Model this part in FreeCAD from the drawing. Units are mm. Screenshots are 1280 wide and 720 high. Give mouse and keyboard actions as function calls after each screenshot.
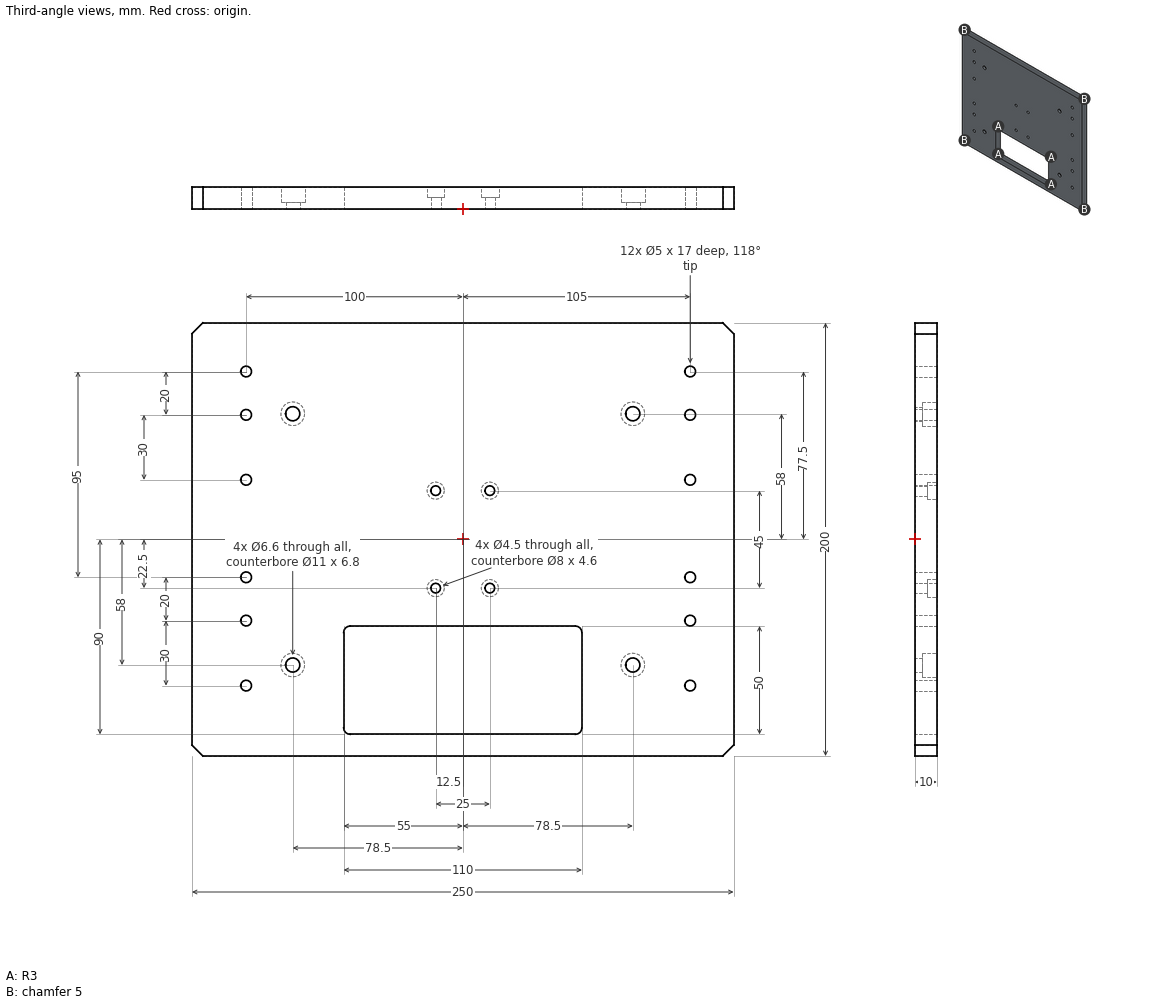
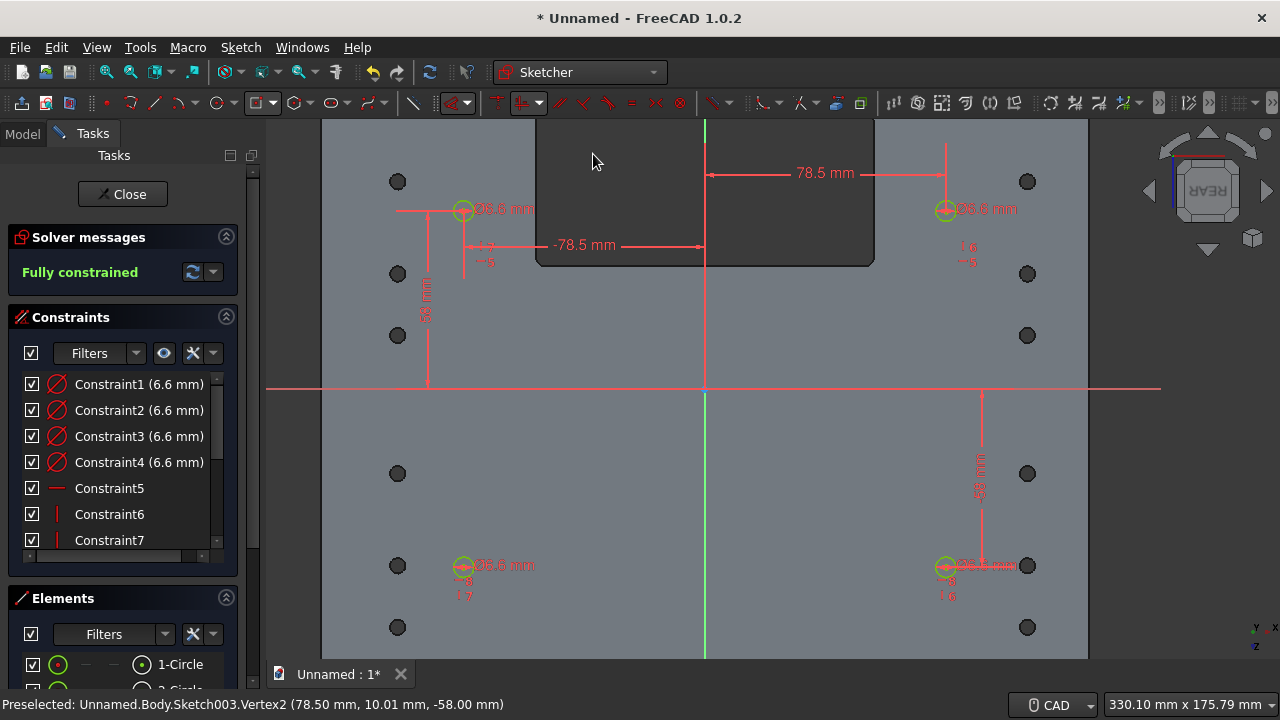
click(123, 194)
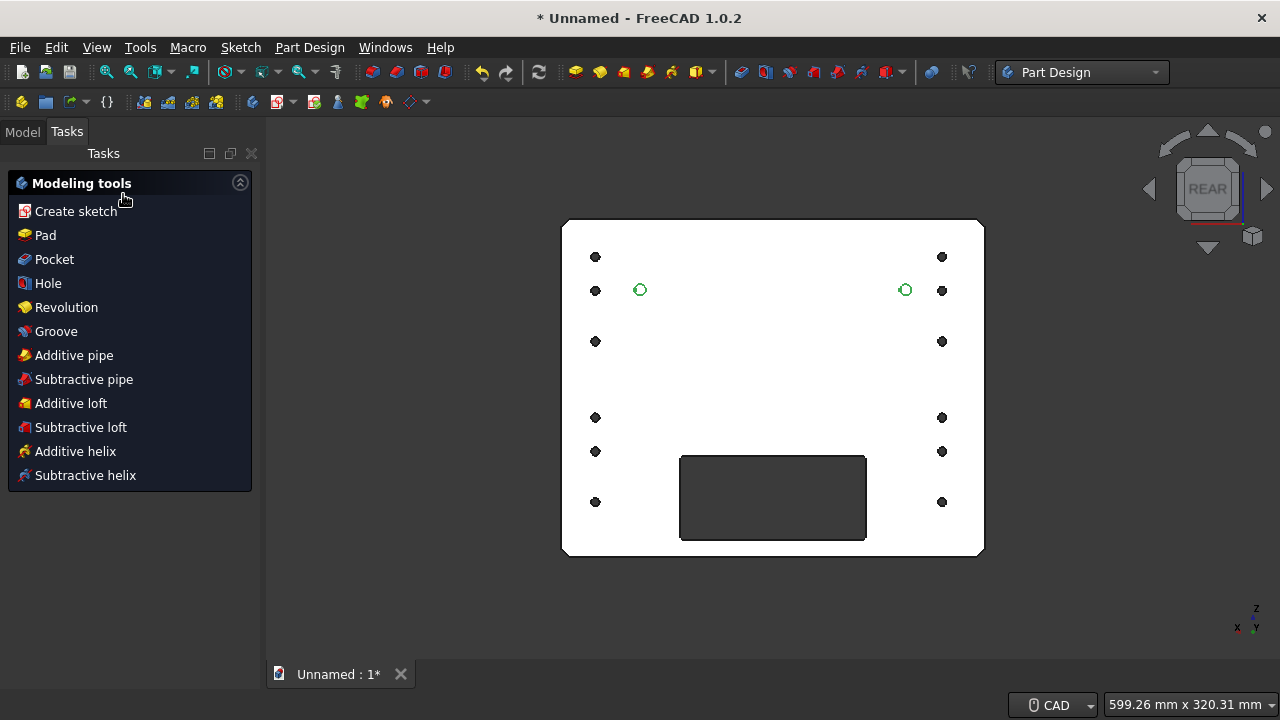
click(766, 72)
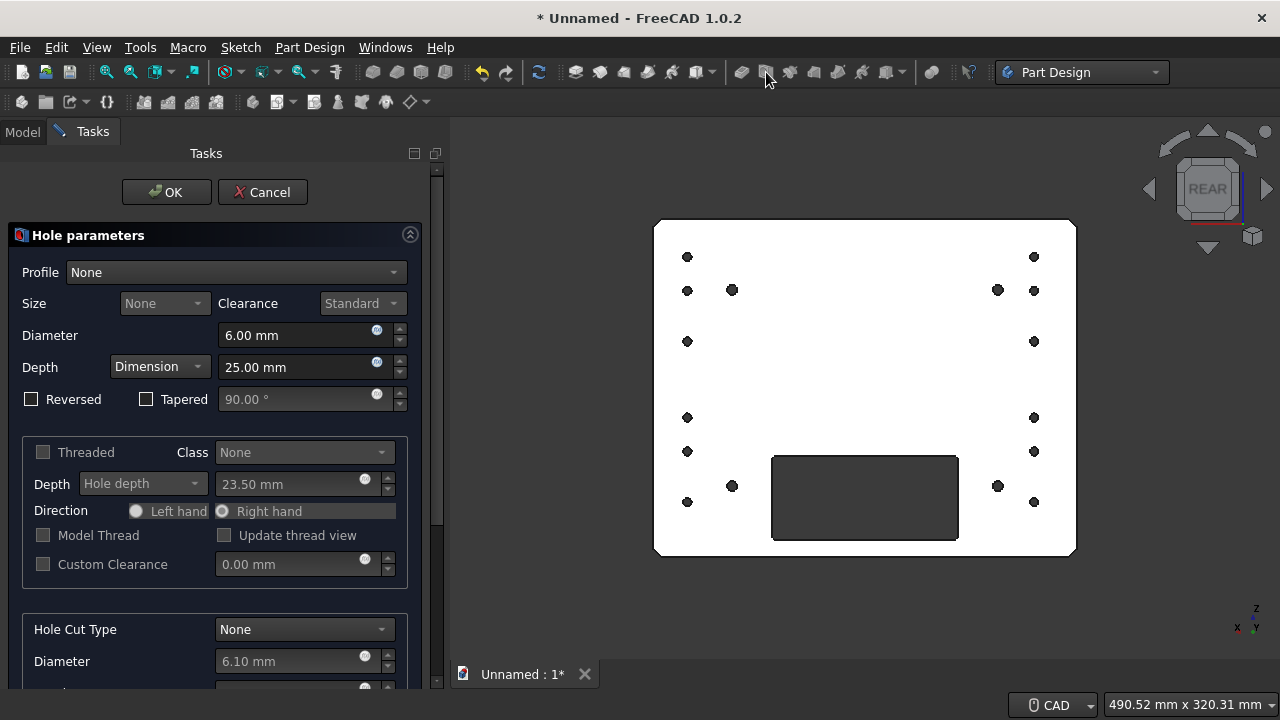
triple_click(305, 335)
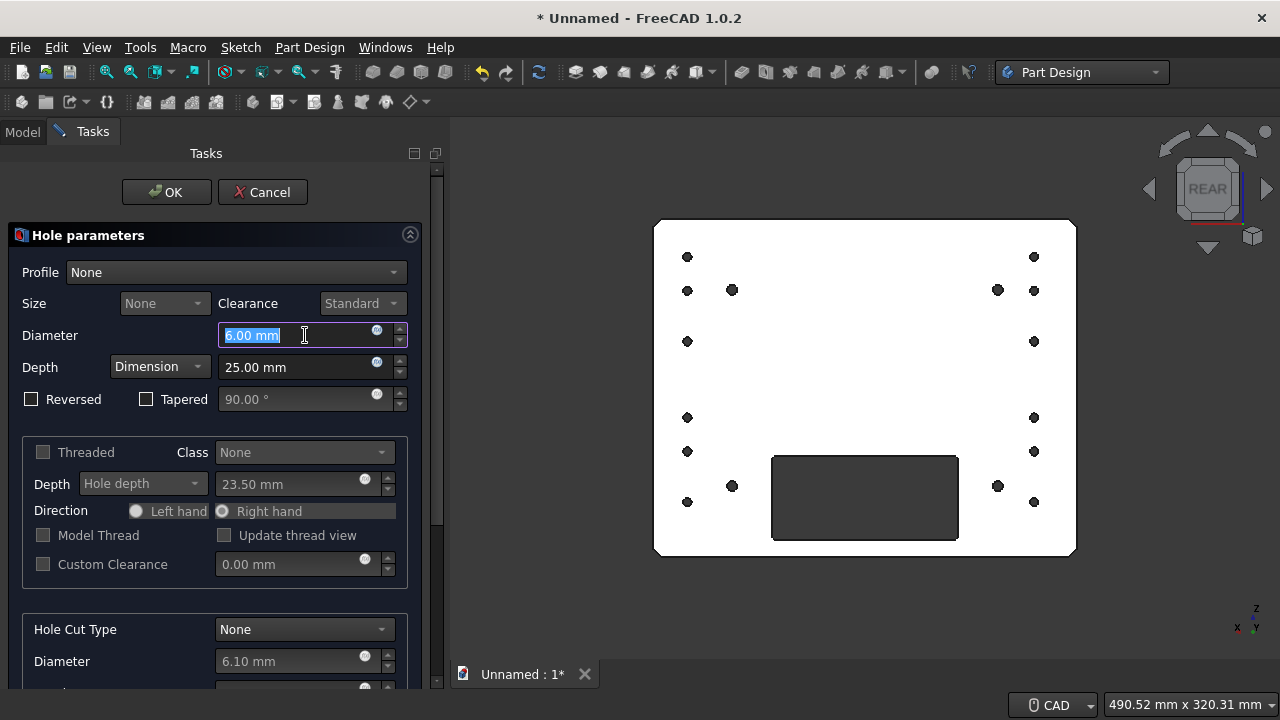
text(6.6)
key(Tab)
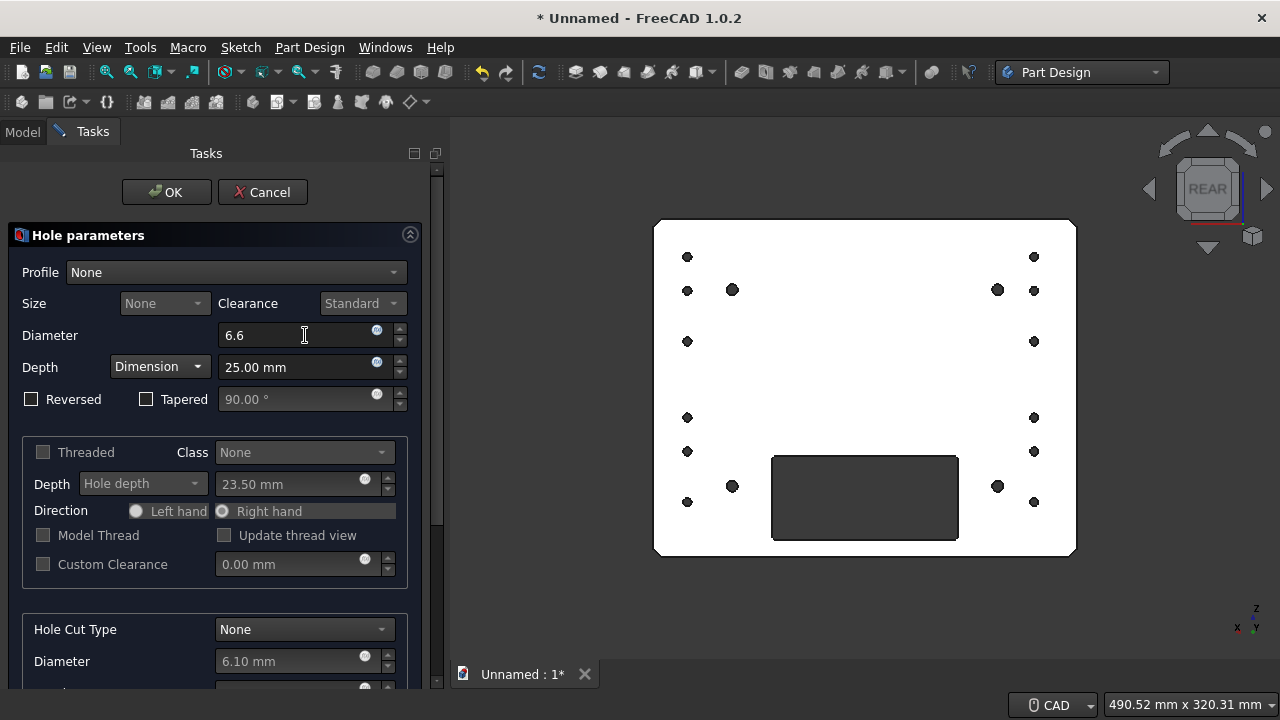
click(161, 366)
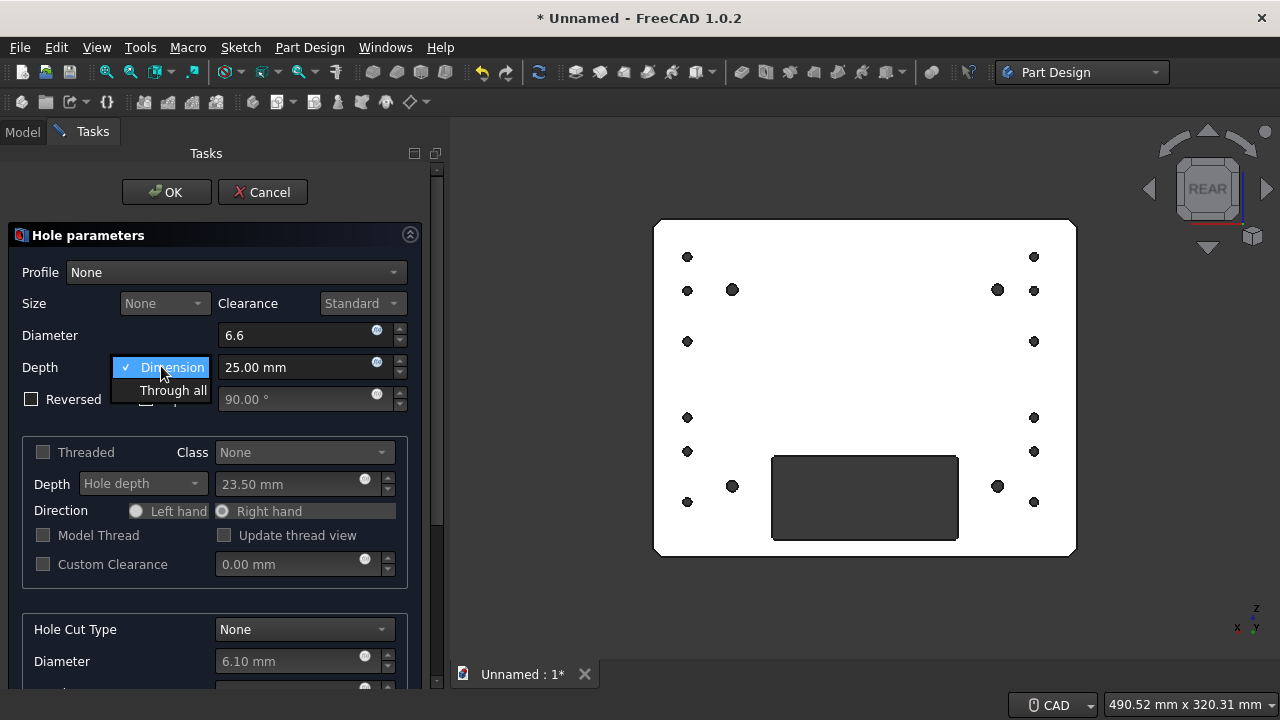
click(160, 390)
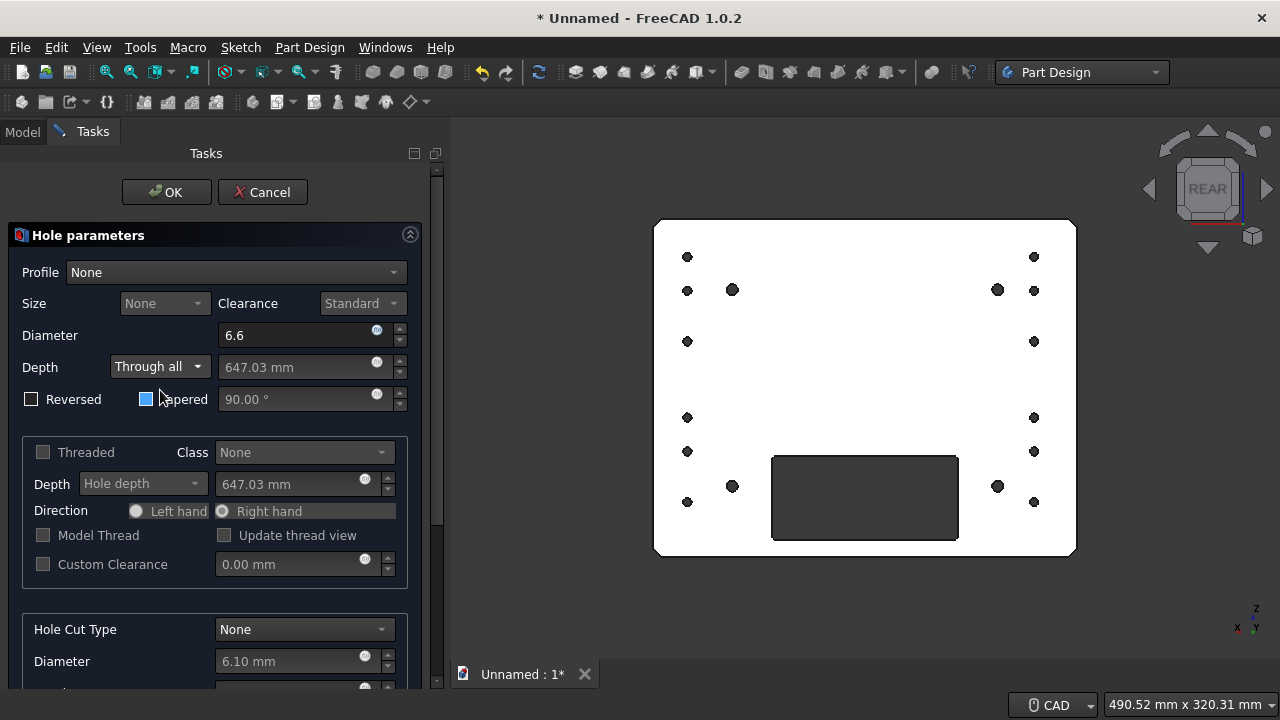
click(306, 630)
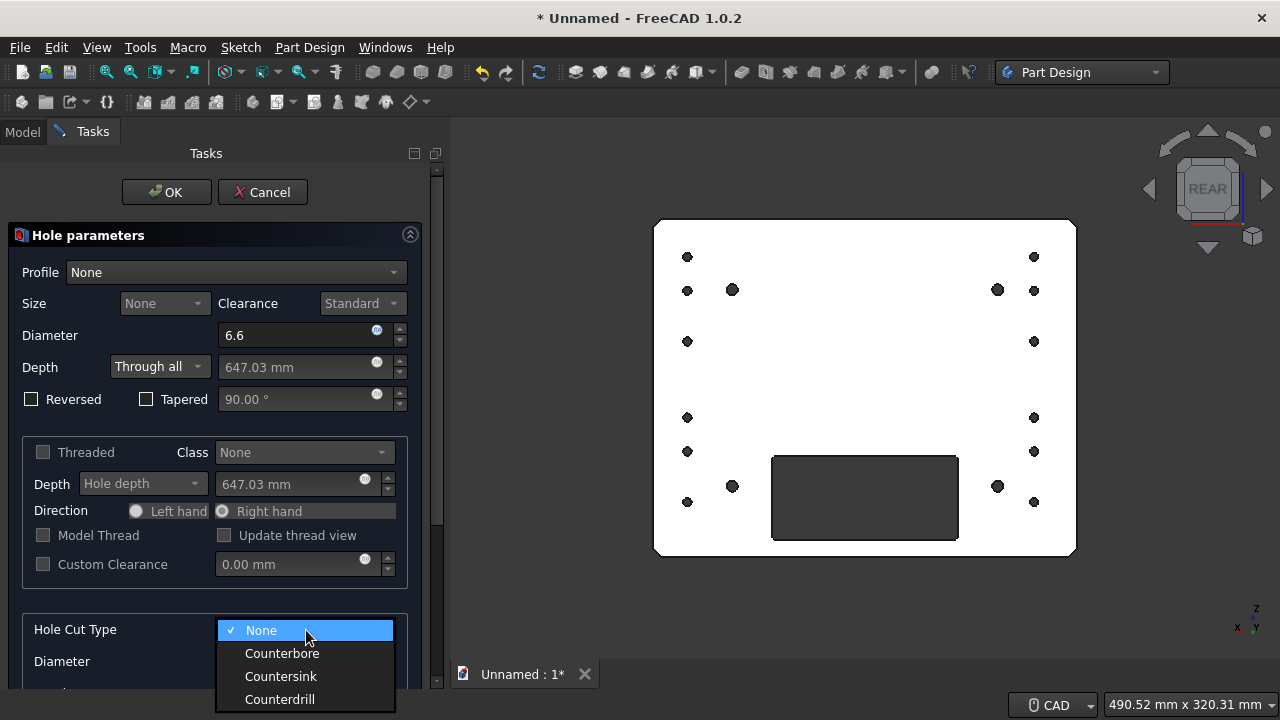
click(304, 654)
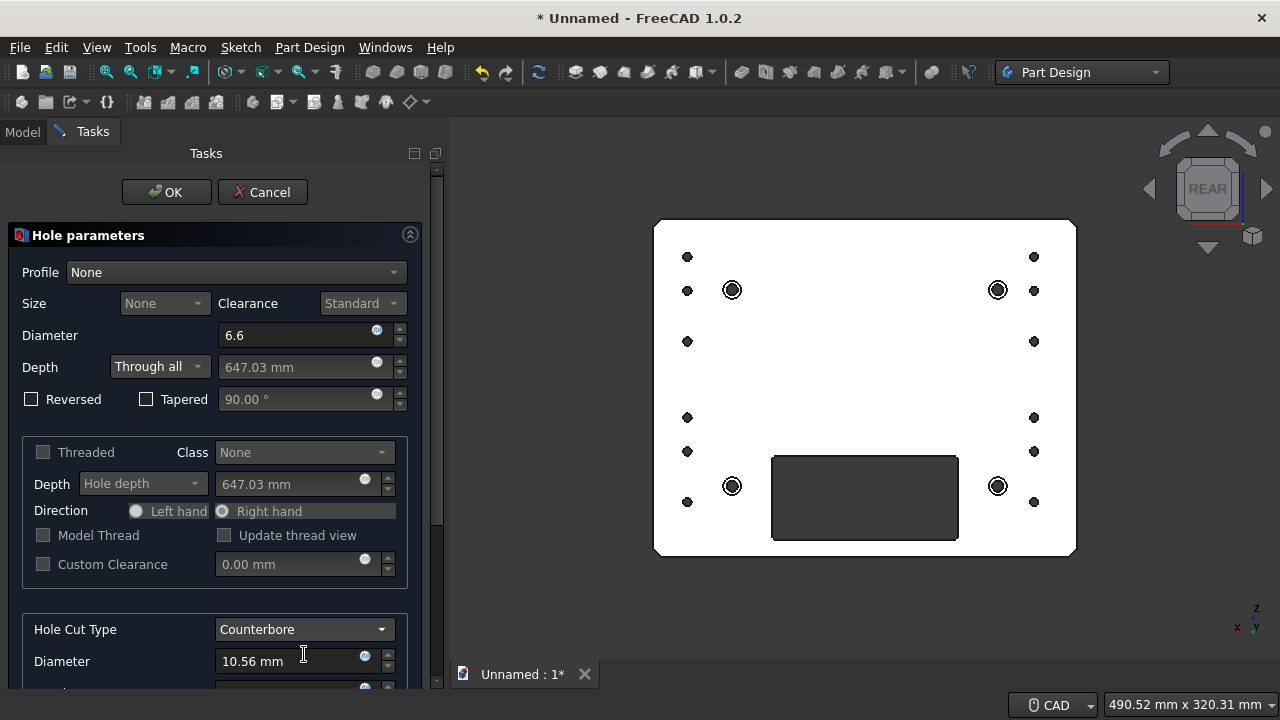
triple_click(298, 661)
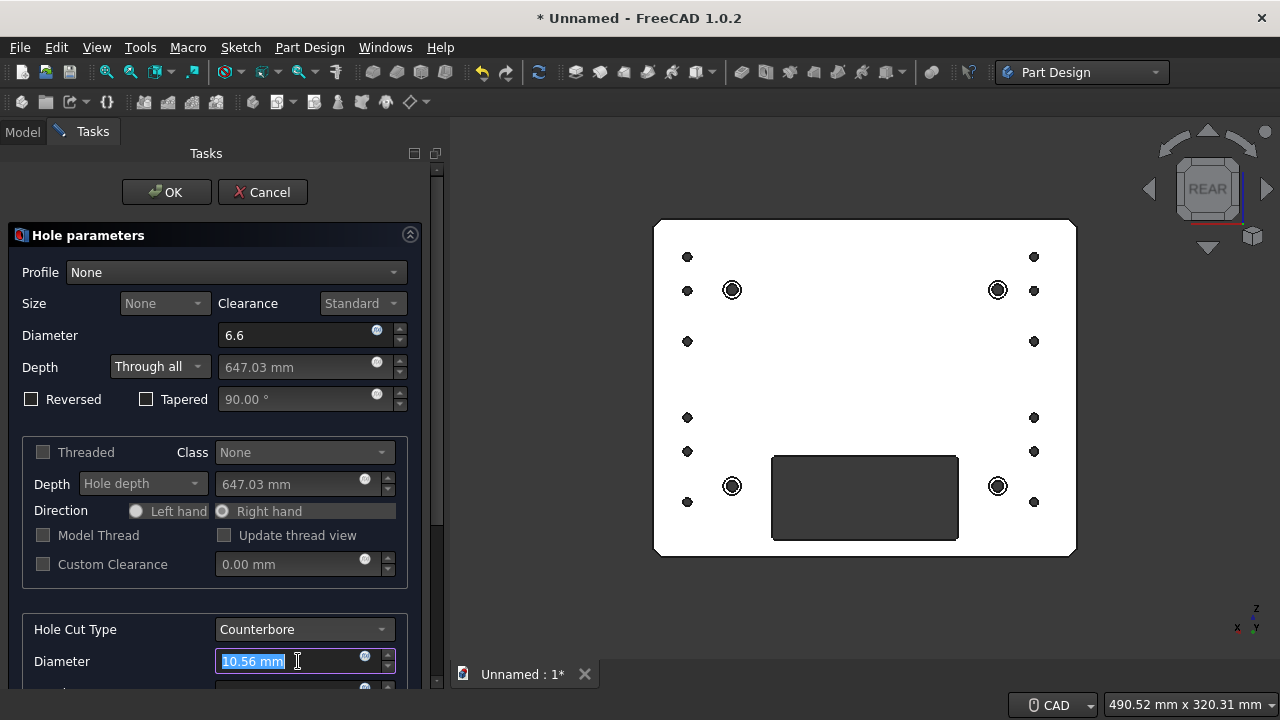
text(11)
key(Tab)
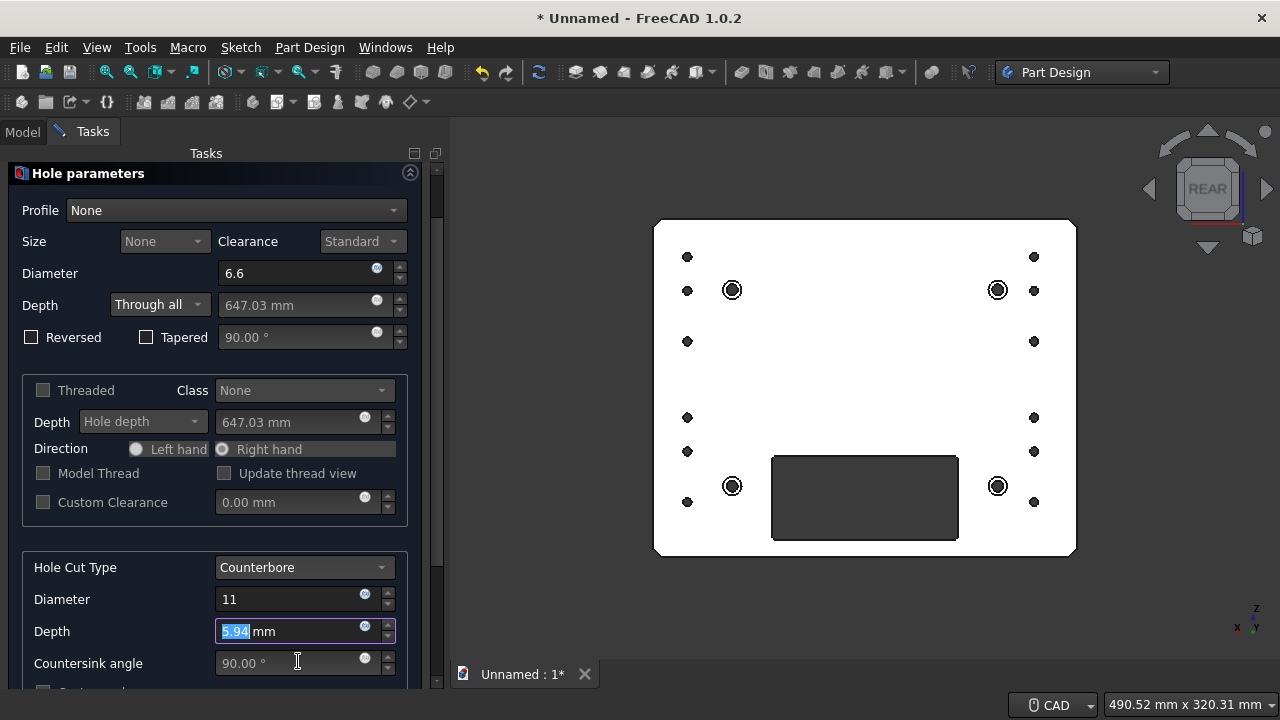
text(6.8)
key(Tab)